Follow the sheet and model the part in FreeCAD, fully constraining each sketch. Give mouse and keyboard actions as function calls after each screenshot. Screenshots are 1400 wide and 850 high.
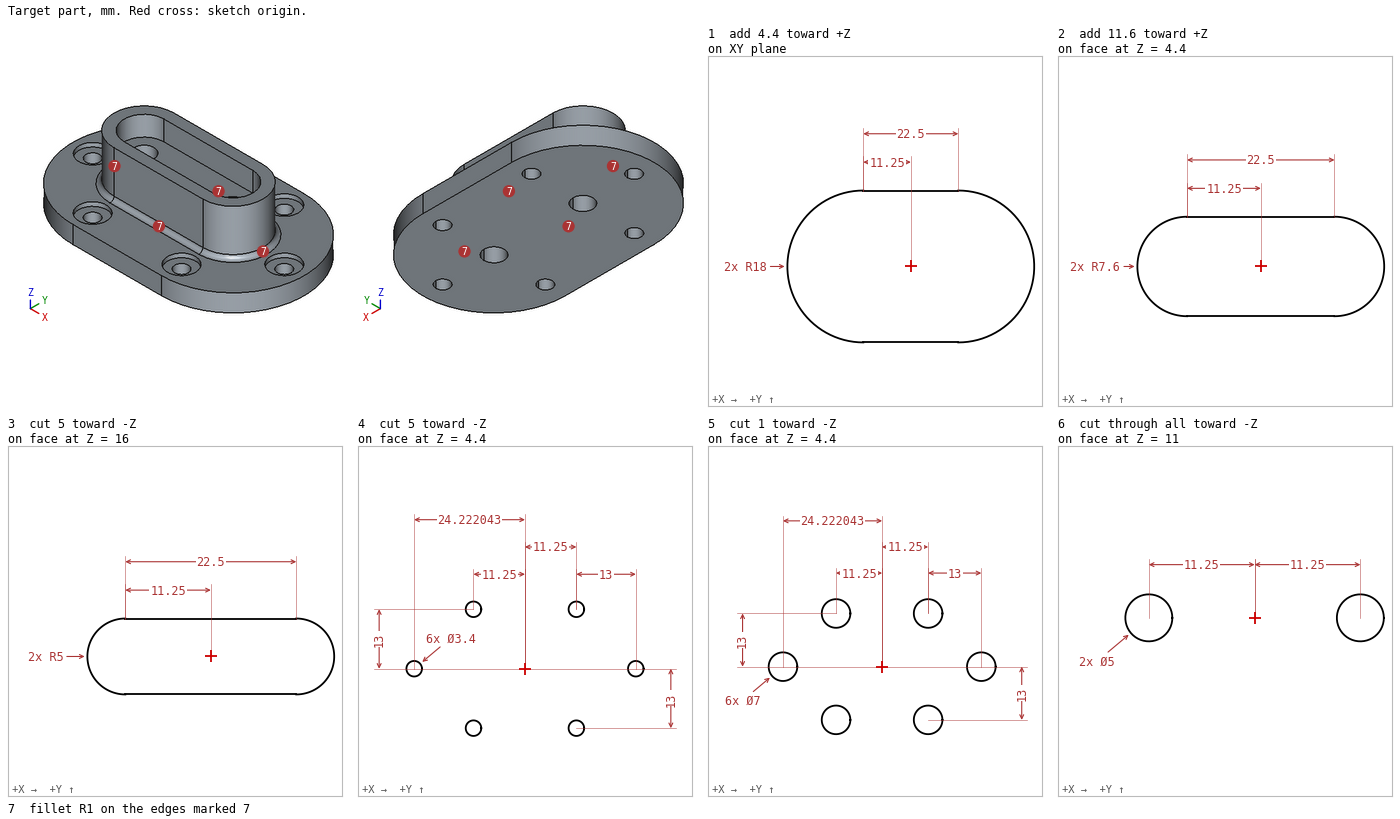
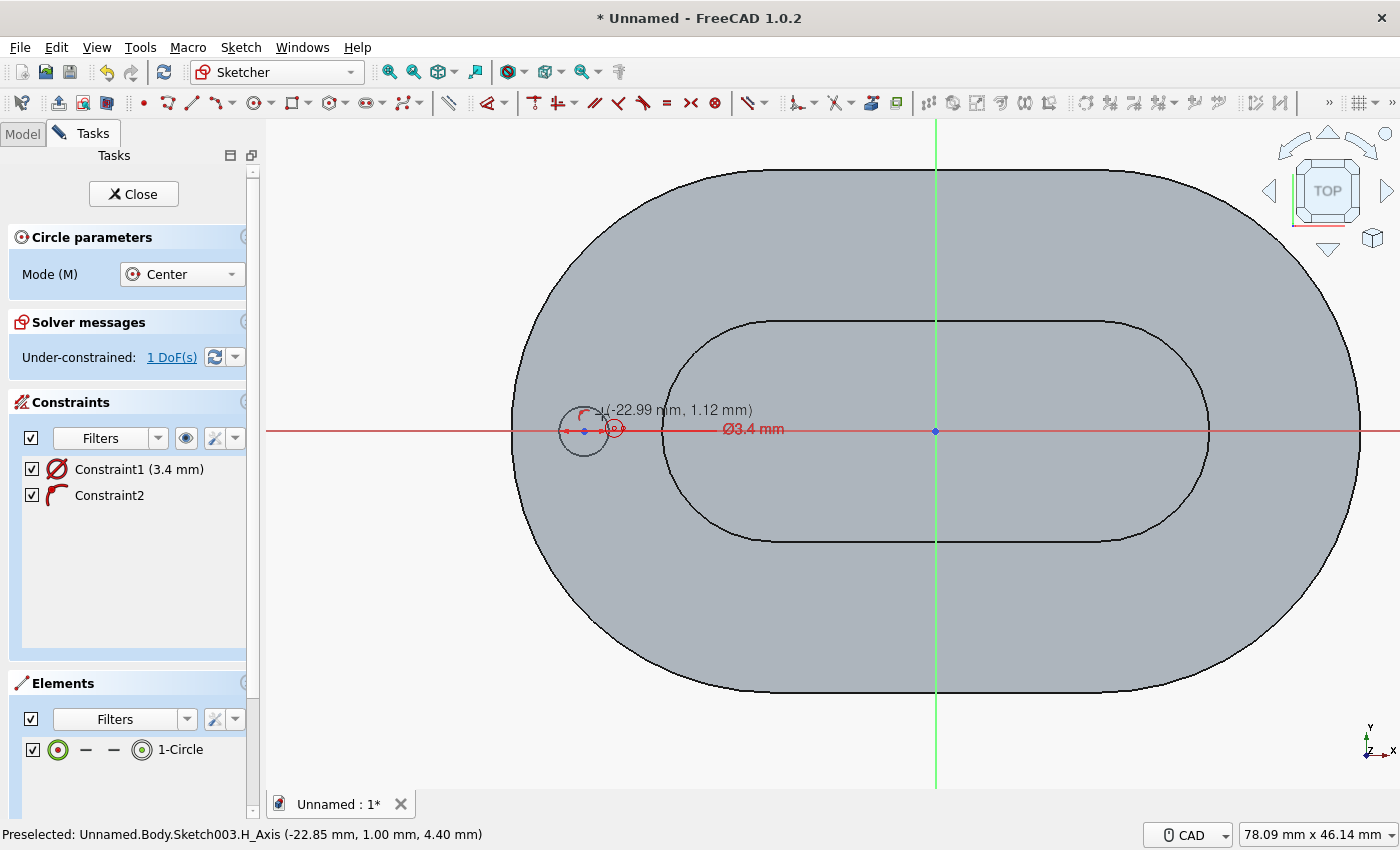
click(772, 242)
move(790, 225)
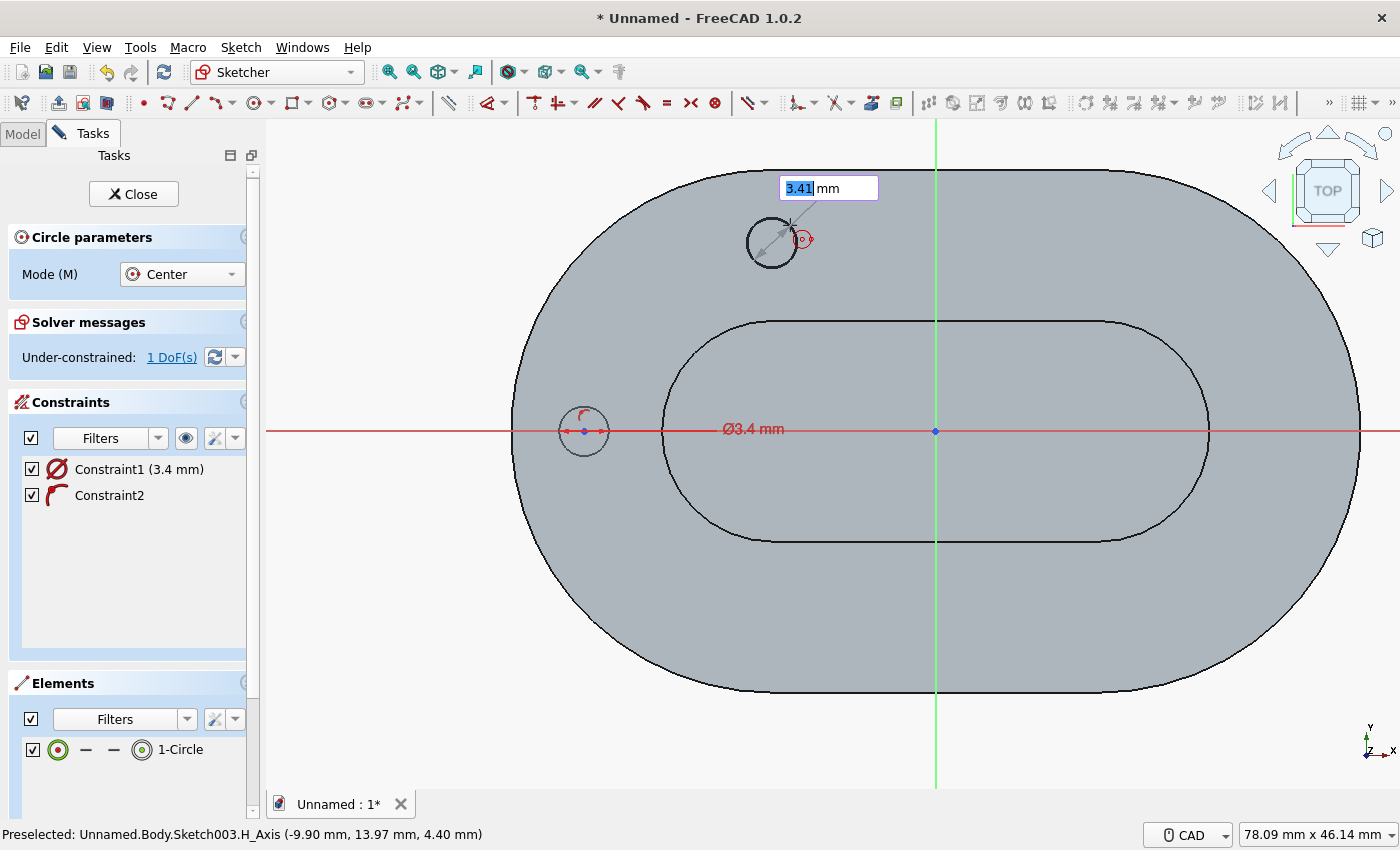
text(3.4)
key(Return)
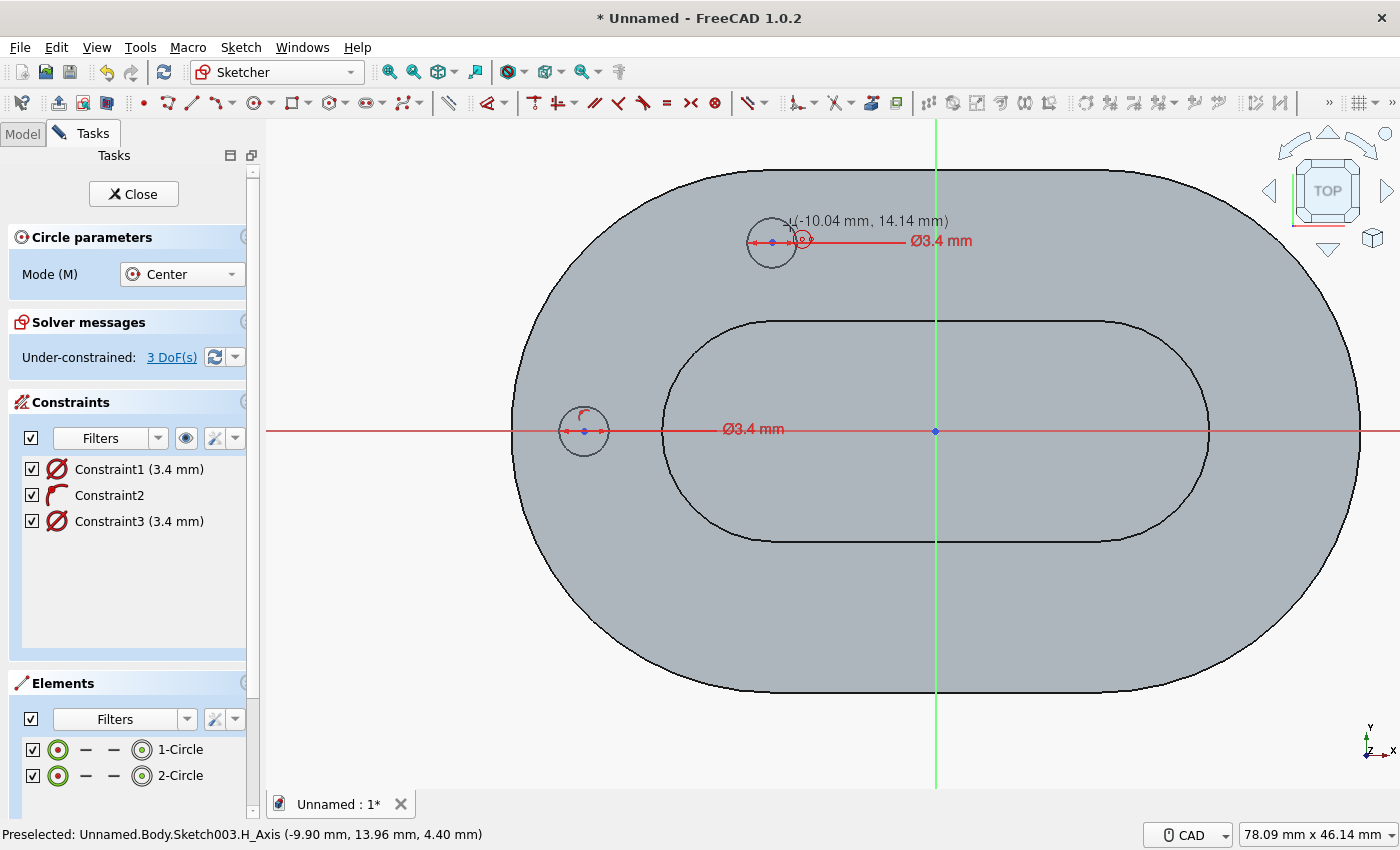
click(1099, 242)
move(1117, 225)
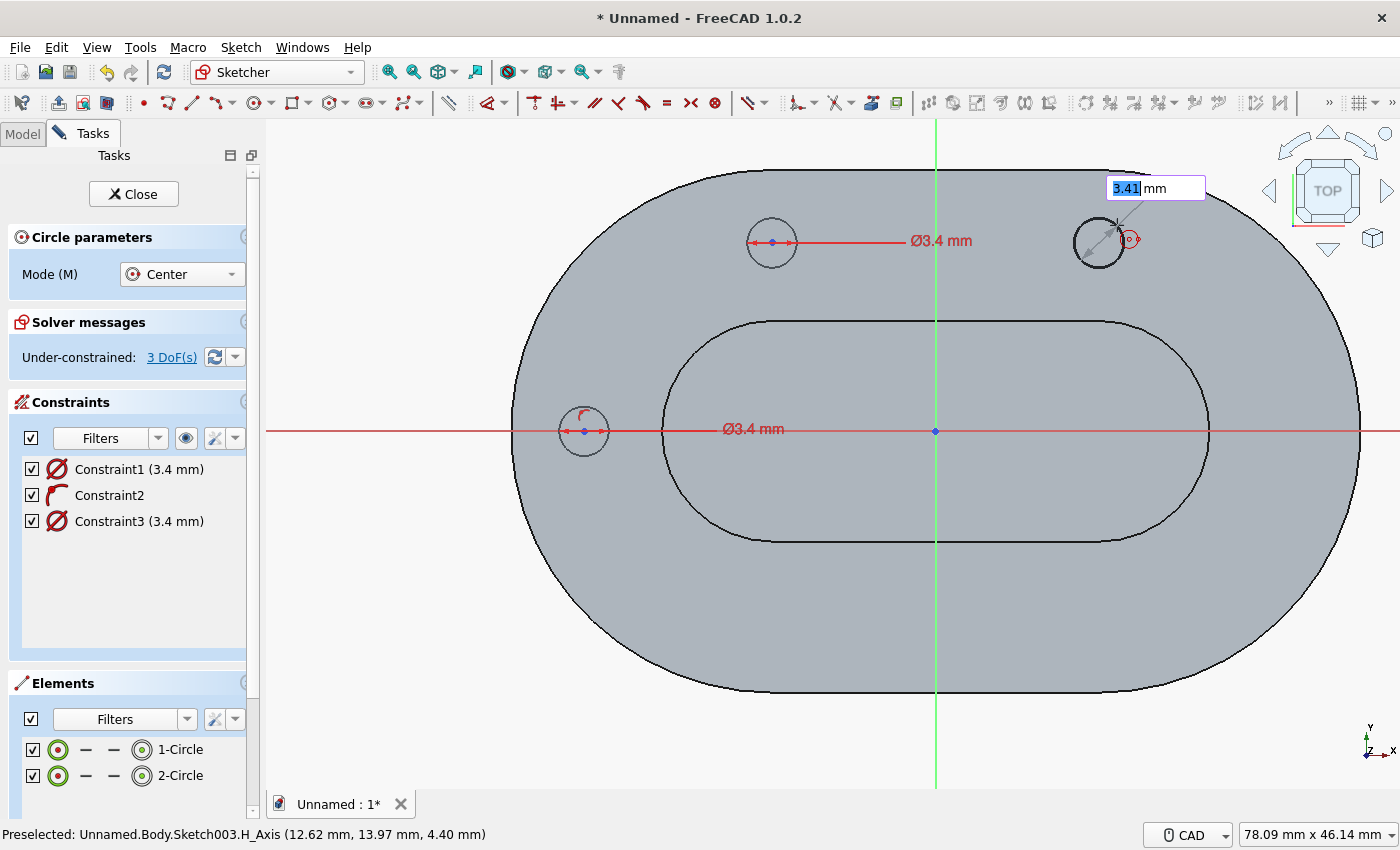
text(3.4)
key(Return)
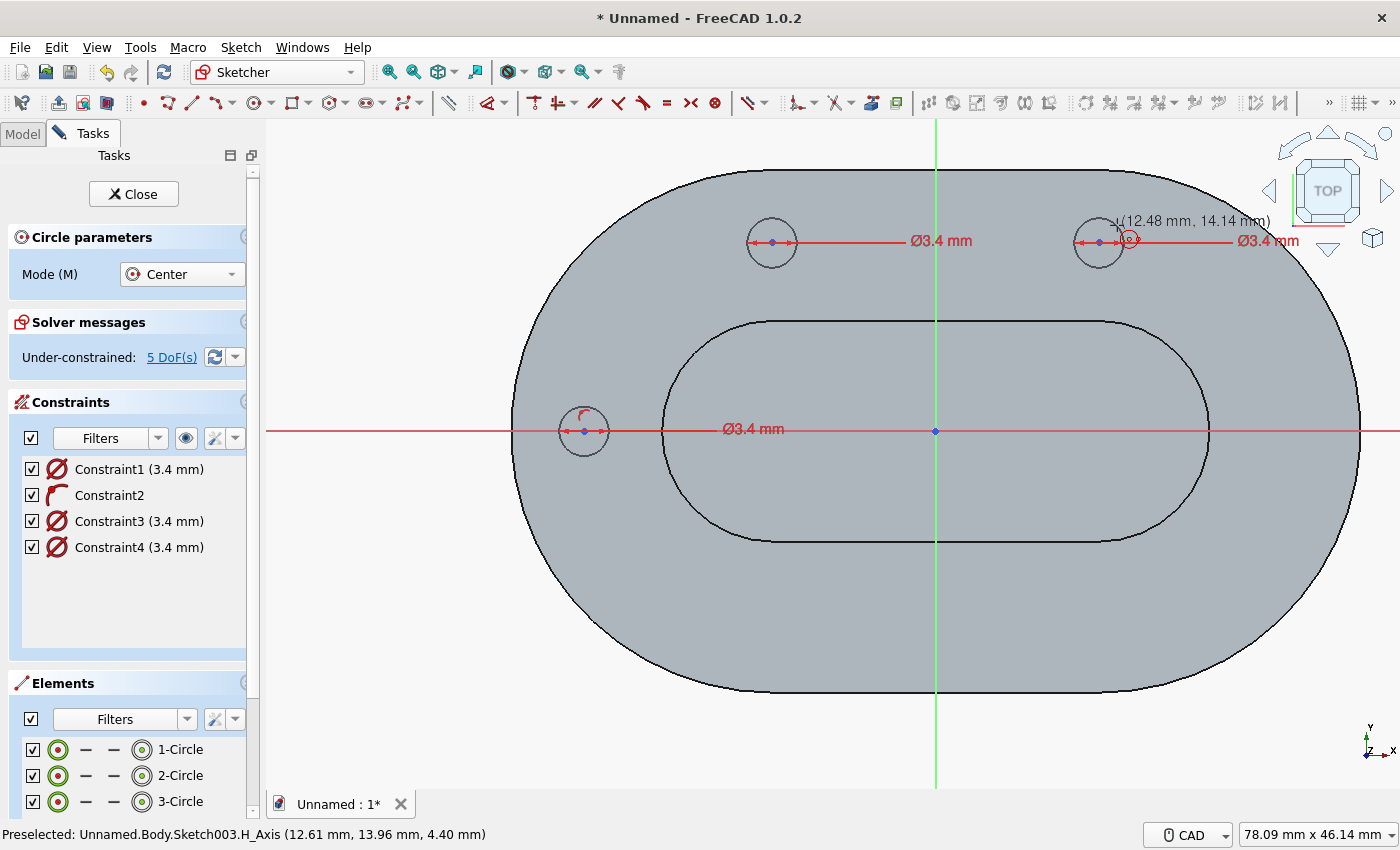
scroll(294, 557, down, 1)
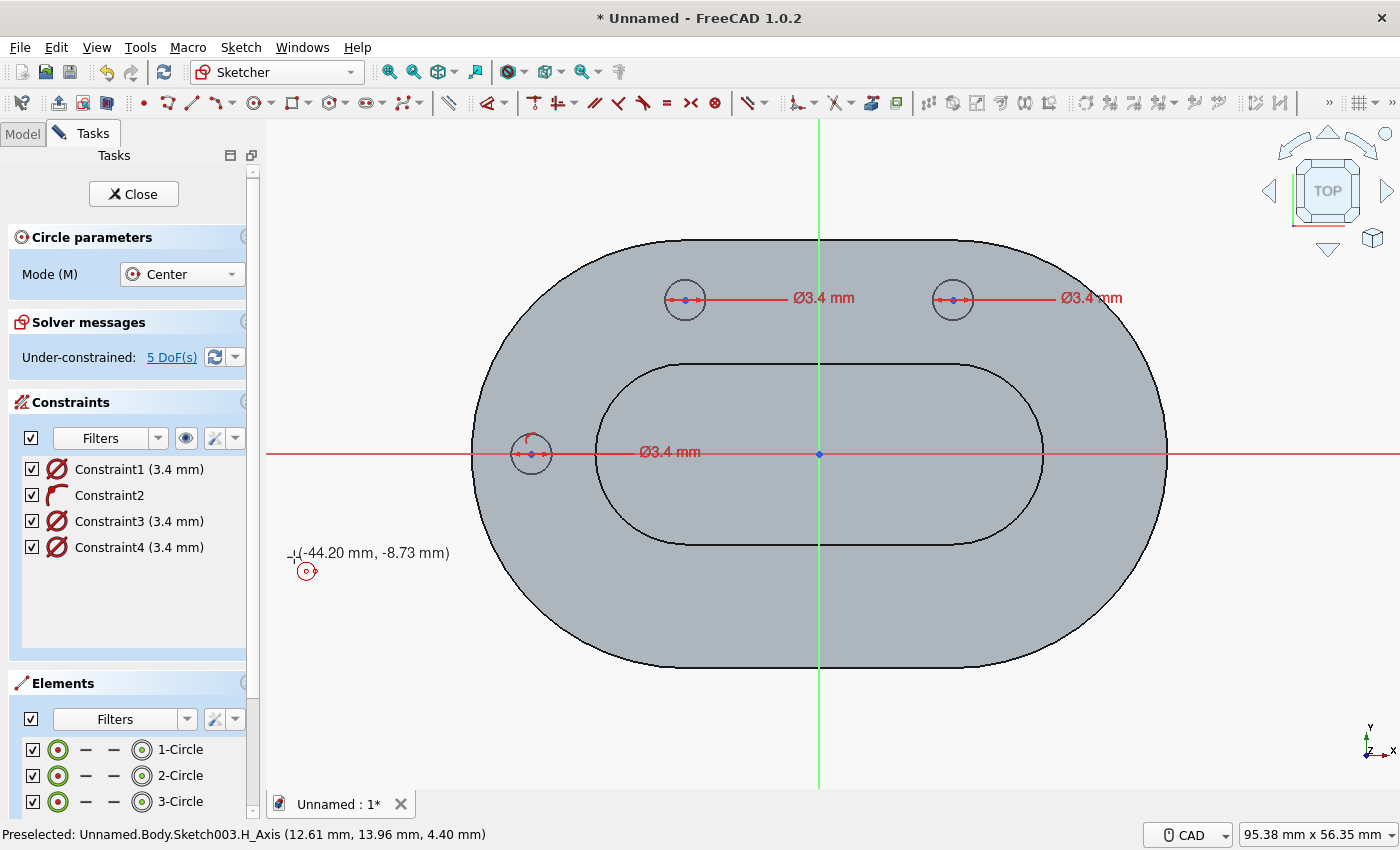
click(1108, 454)
move(1122, 440)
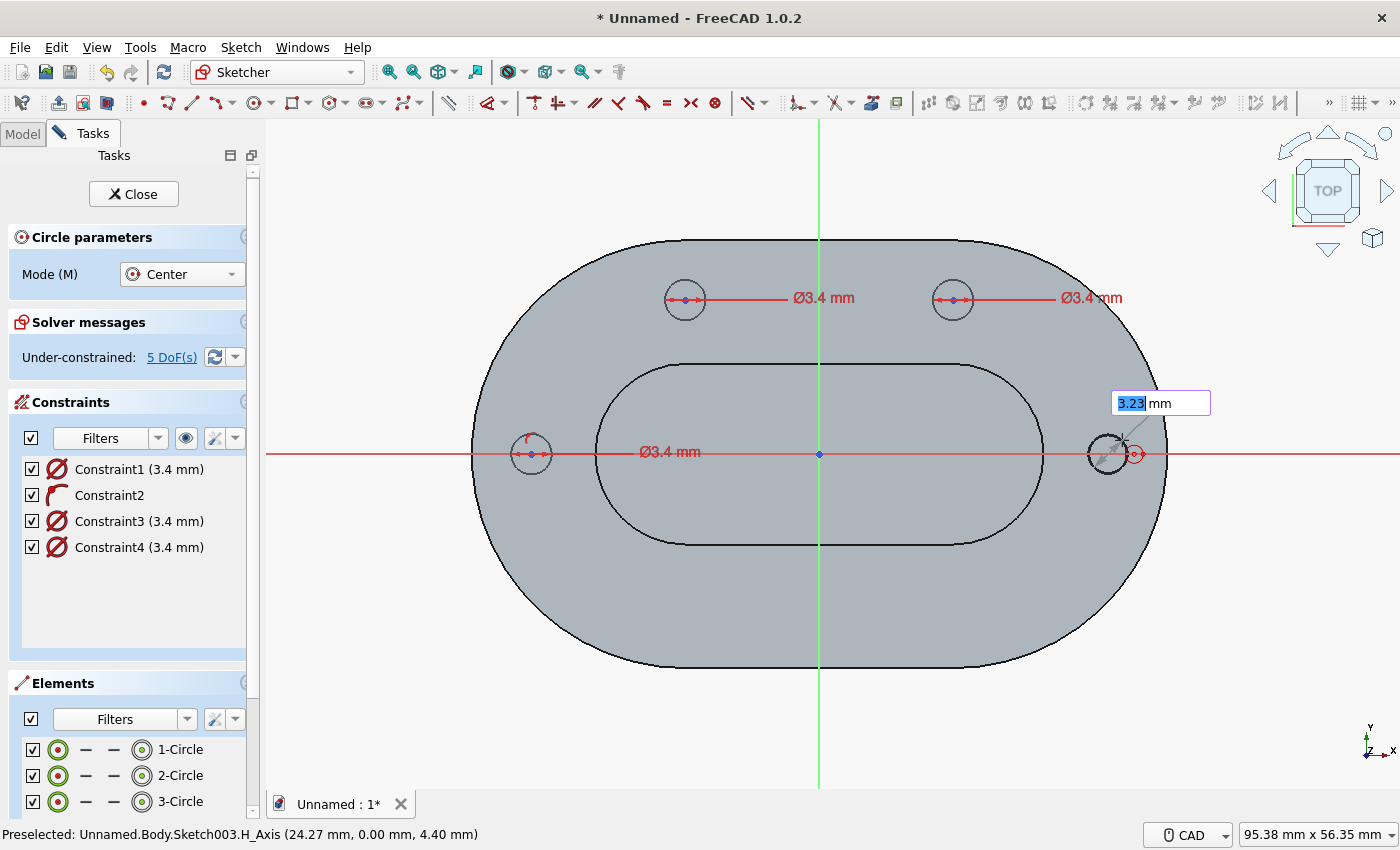
text(3.4)
key(Return)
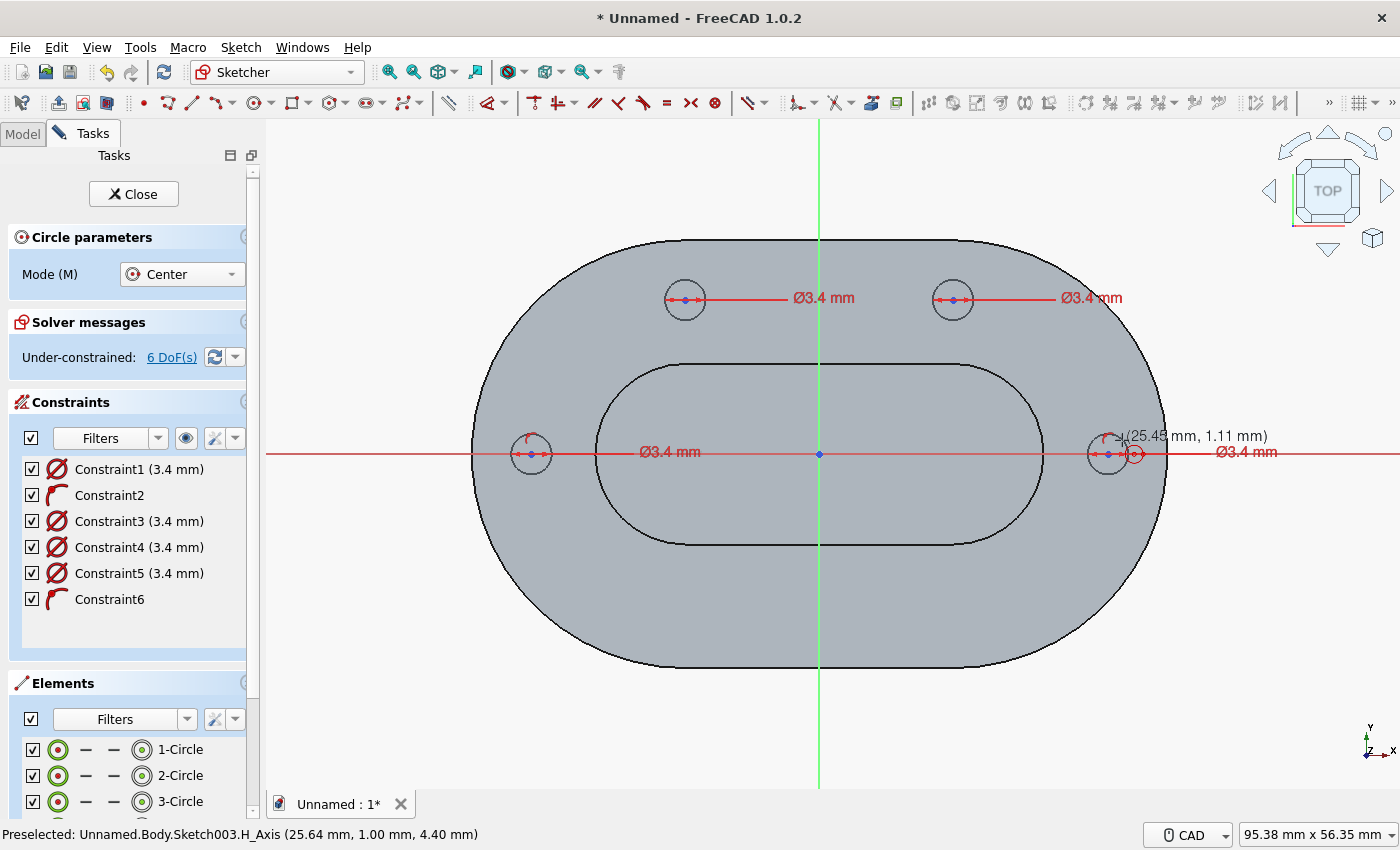
click(953, 609)
move(968, 594)